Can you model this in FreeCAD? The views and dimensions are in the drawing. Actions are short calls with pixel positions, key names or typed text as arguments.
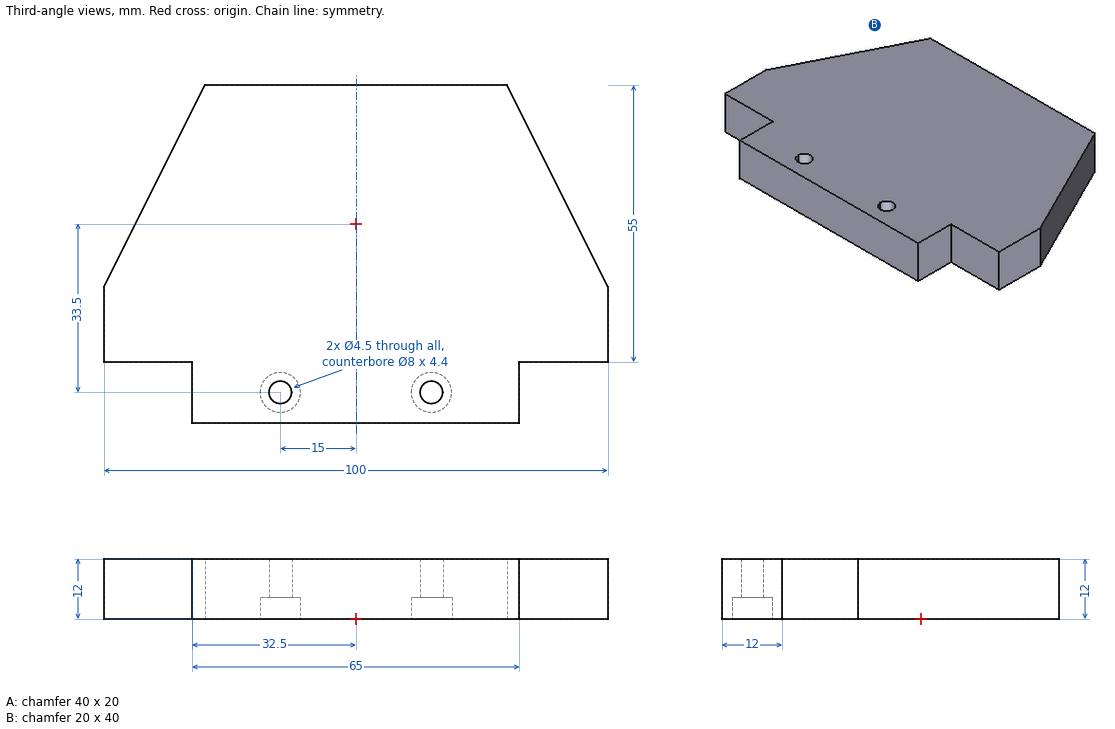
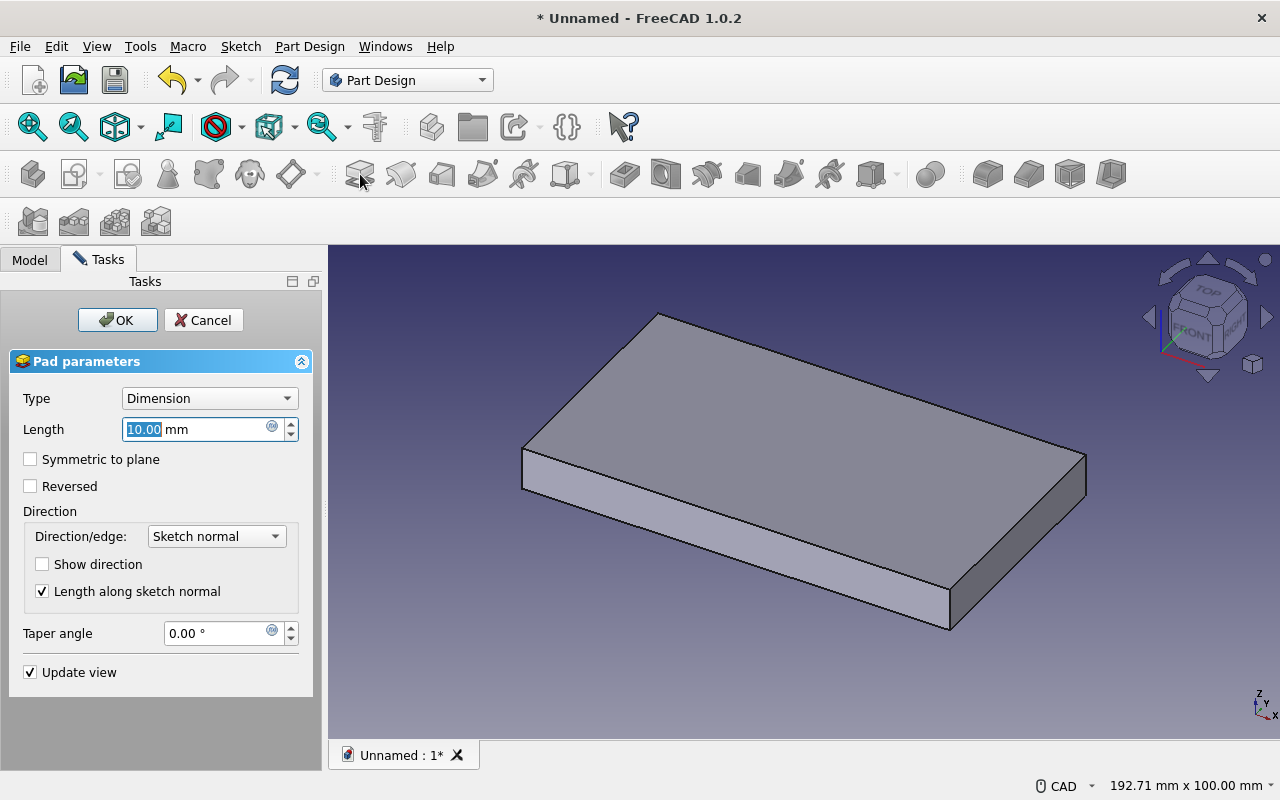
text(12)
key(Tab)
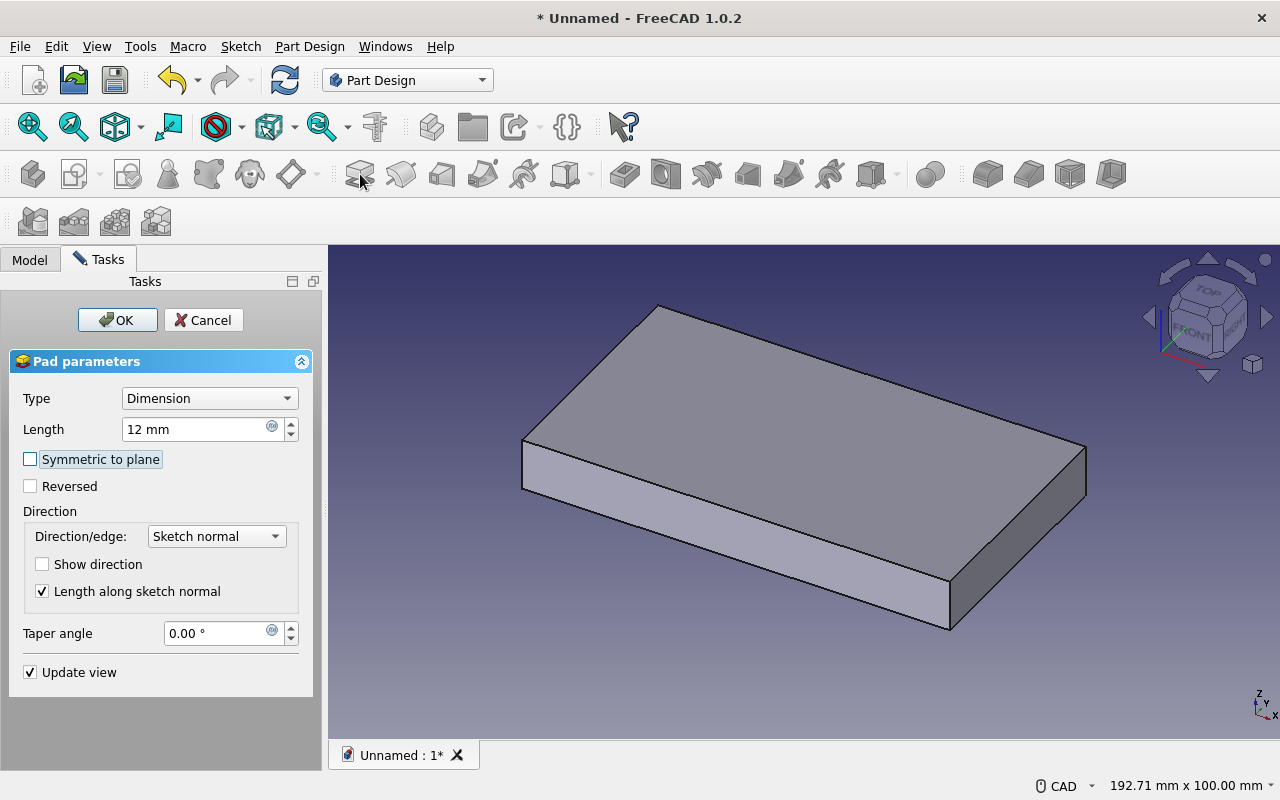
click(118, 320)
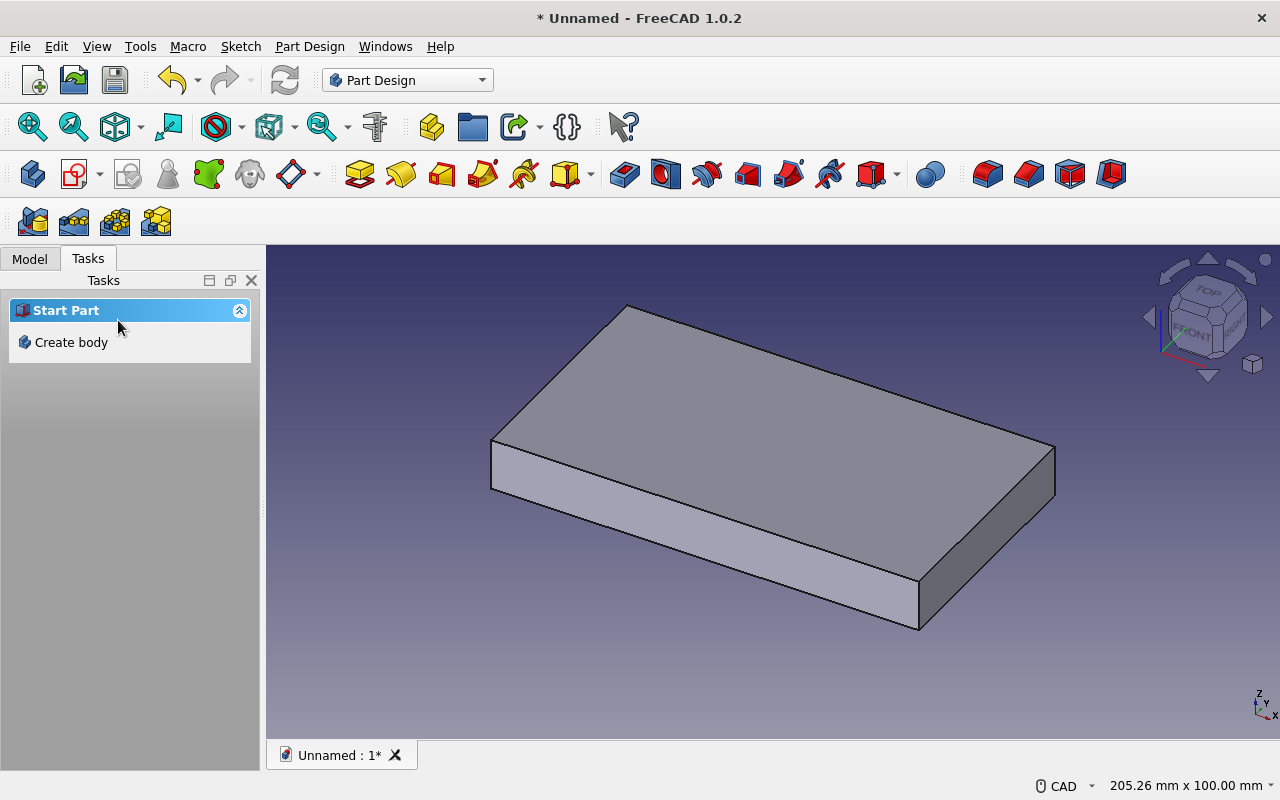
click(888, 595)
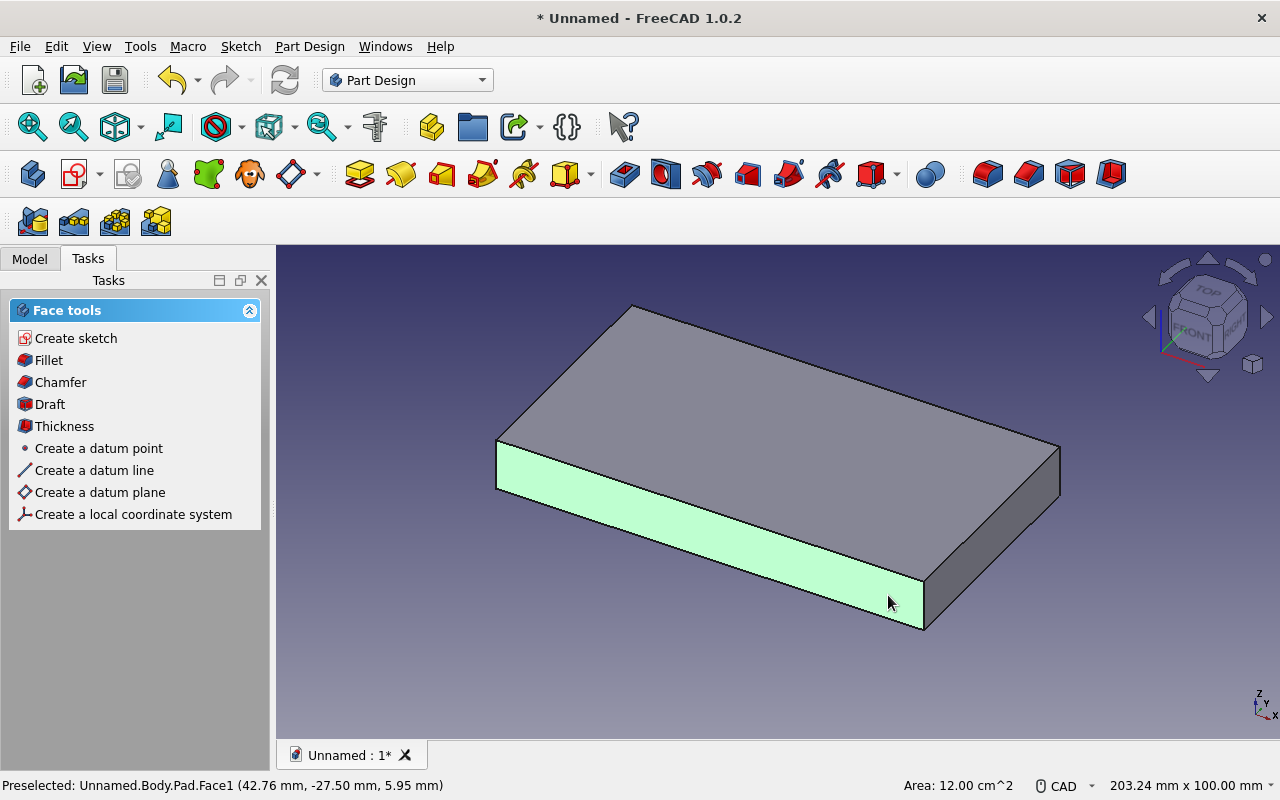
click(74, 174)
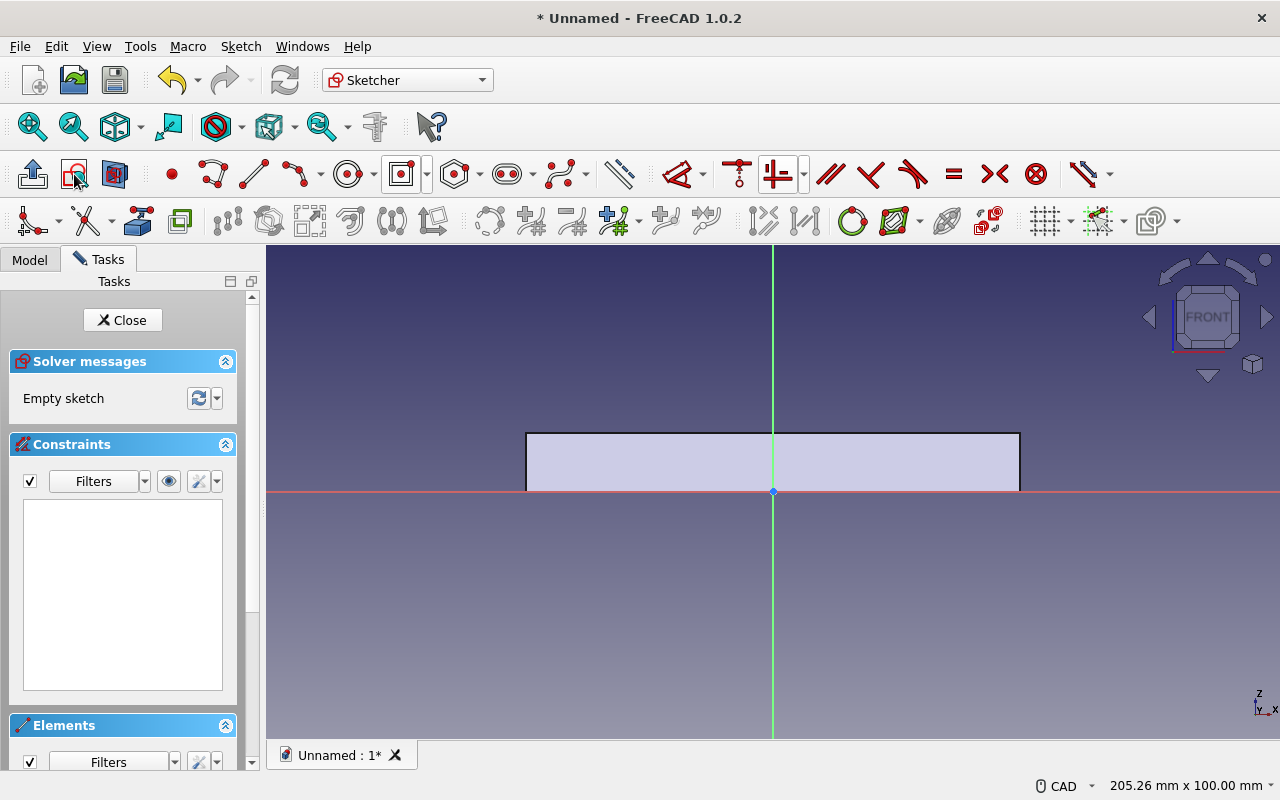
scroll(856, 426, up, 3)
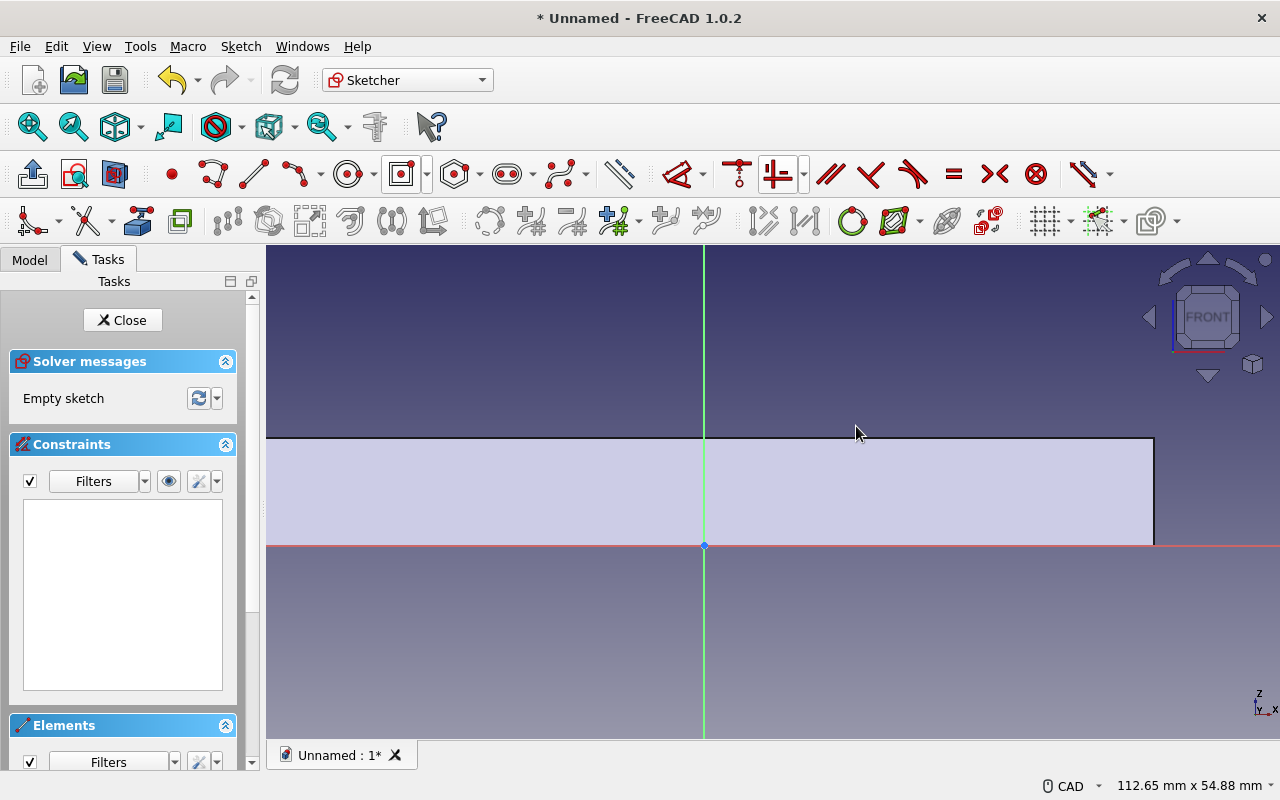
key(g)
key(r)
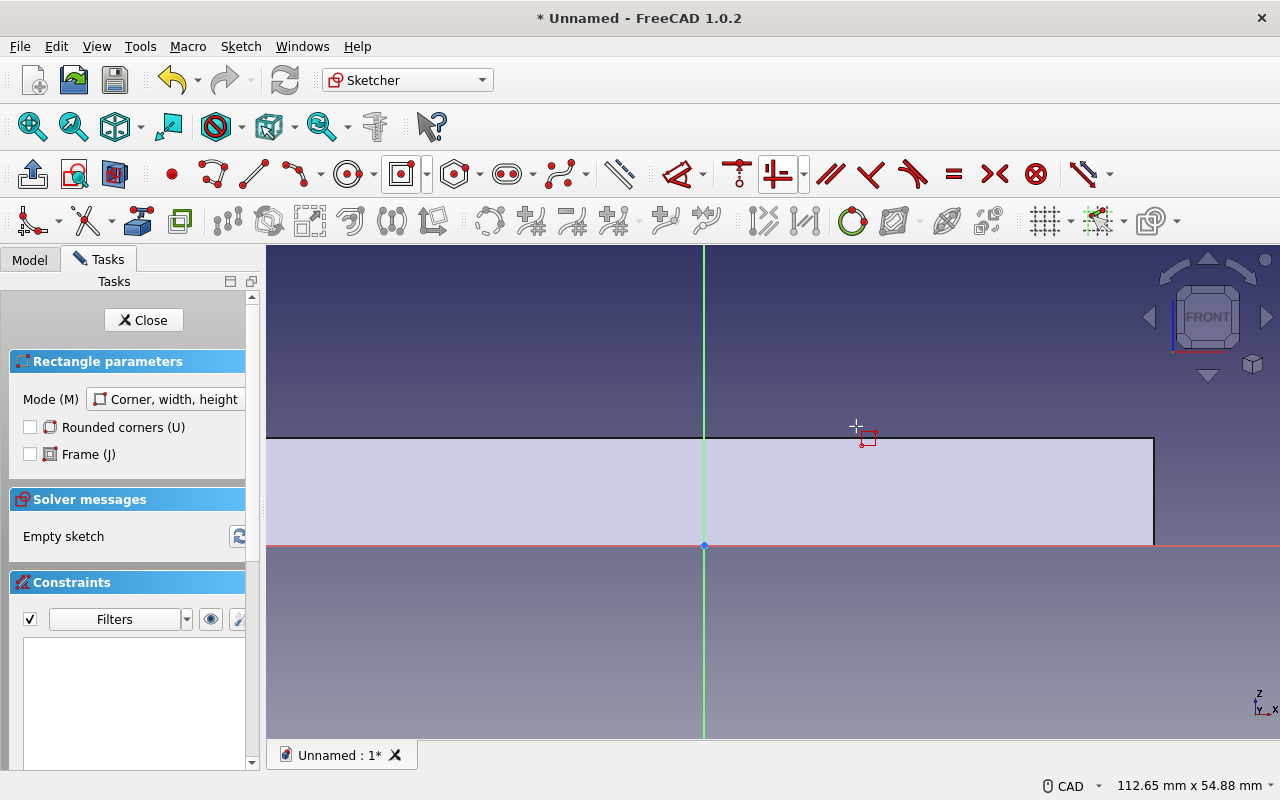
click(412, 438)
click(997, 546)
key(Escape)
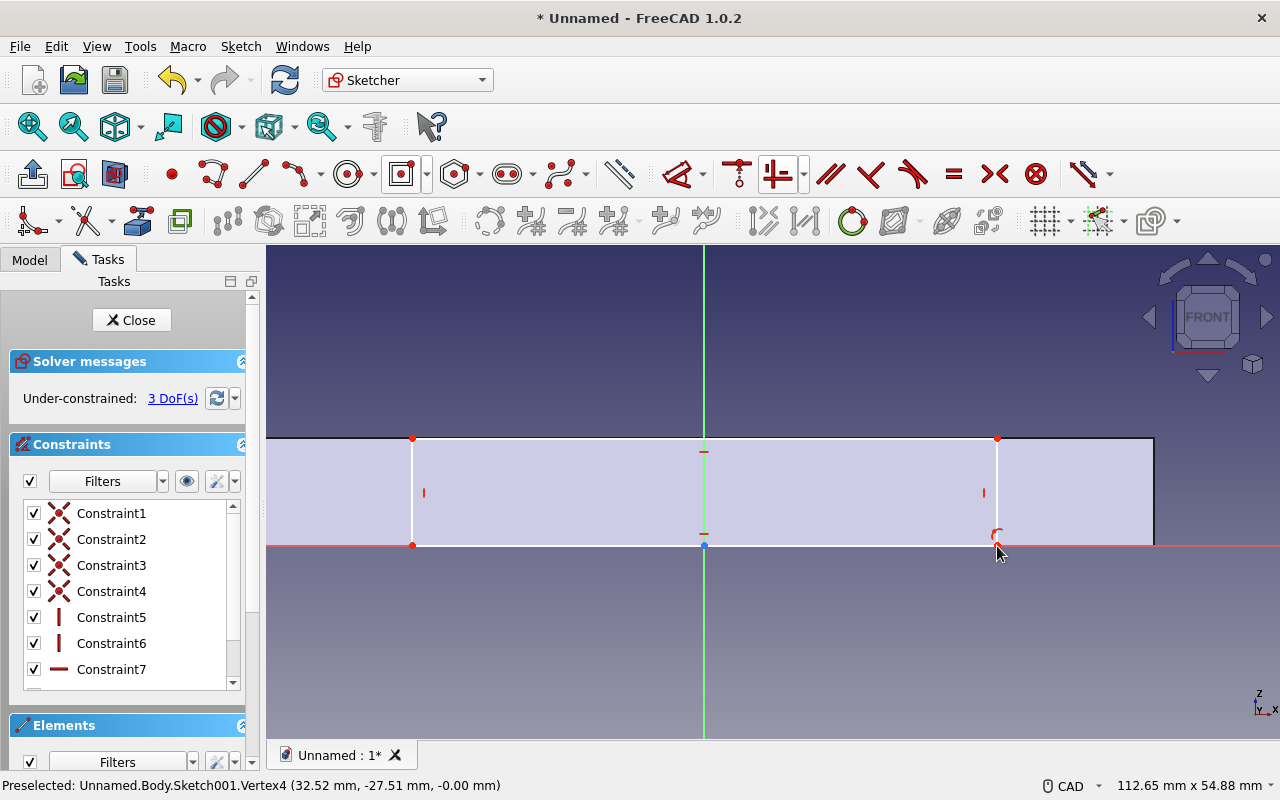
click(676, 174)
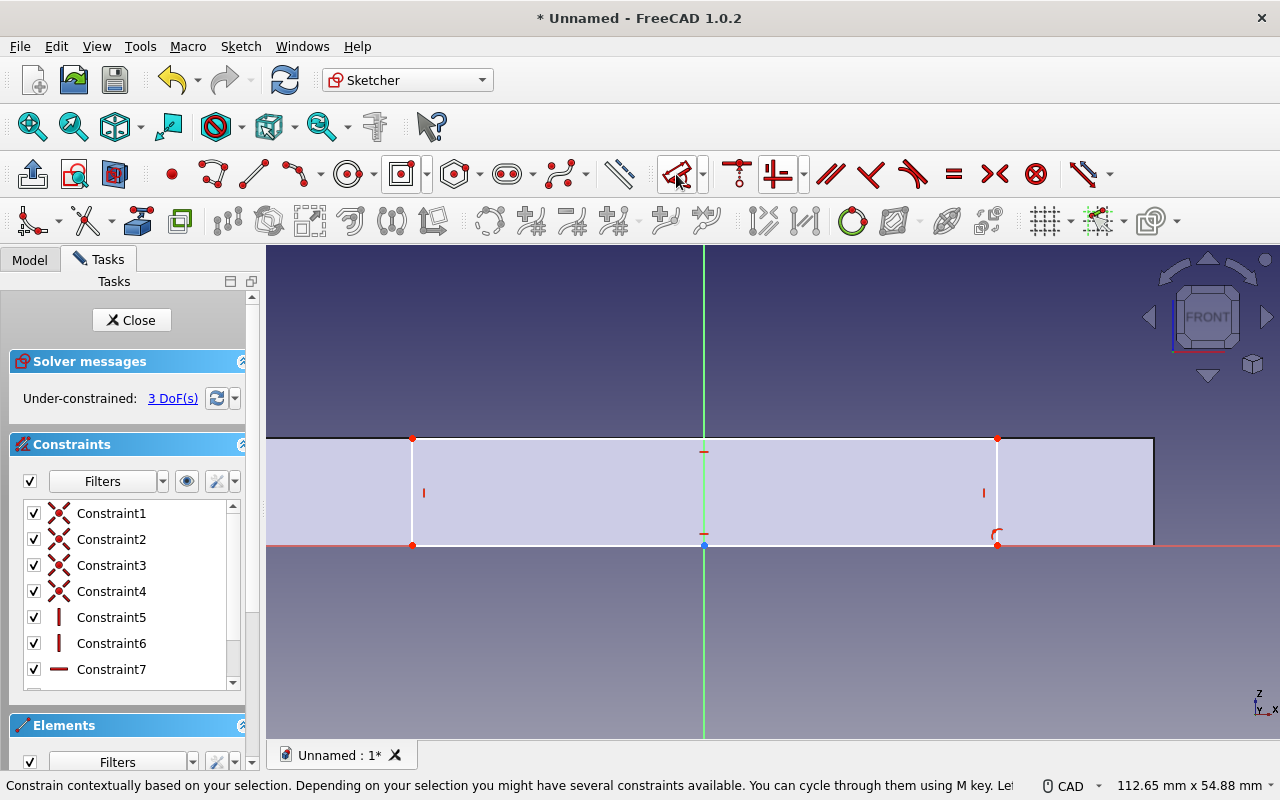
click(412, 471)
click(378, 492)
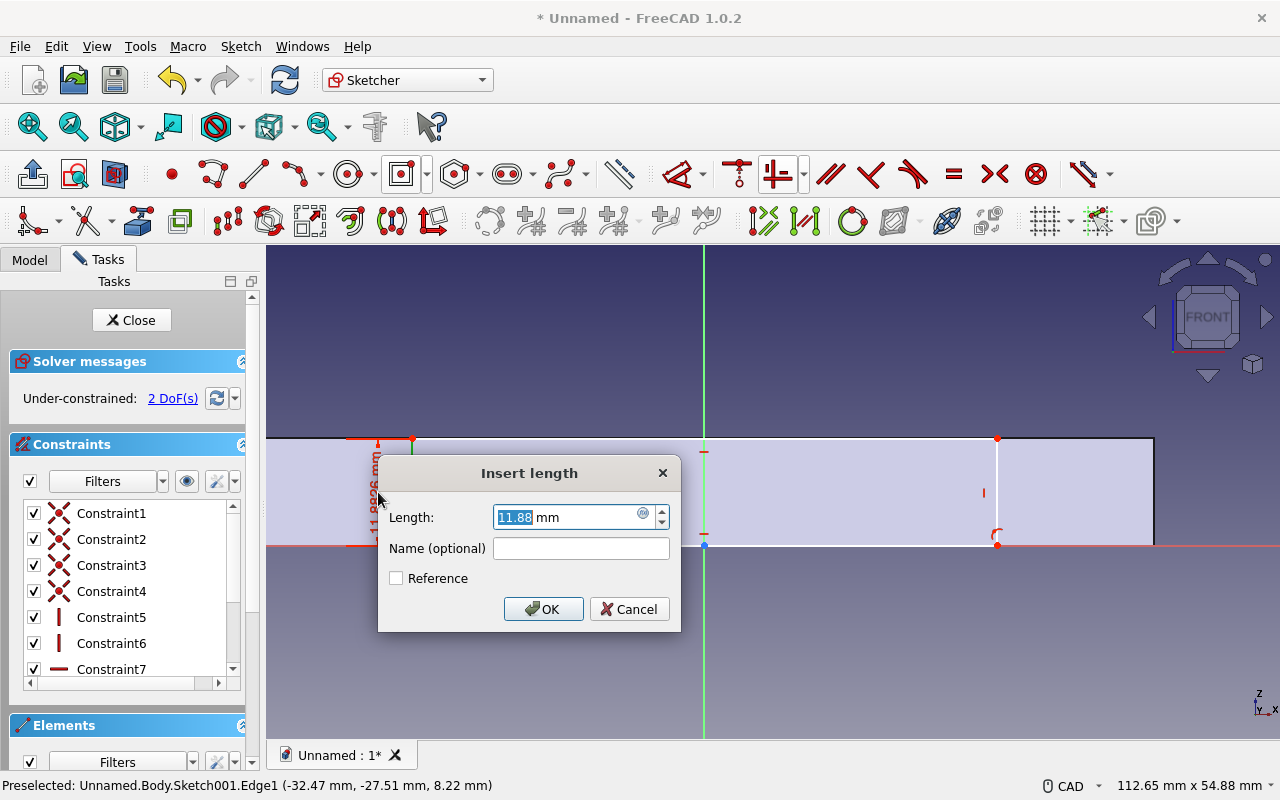
text(12)
key(Return)